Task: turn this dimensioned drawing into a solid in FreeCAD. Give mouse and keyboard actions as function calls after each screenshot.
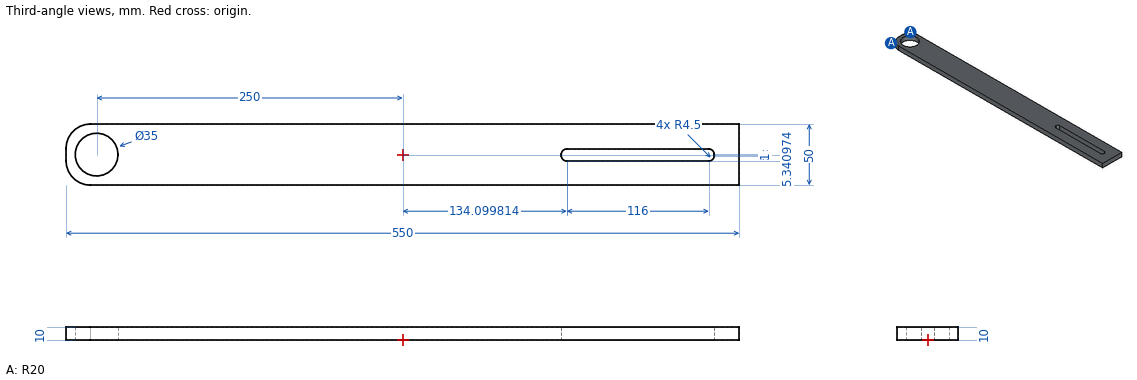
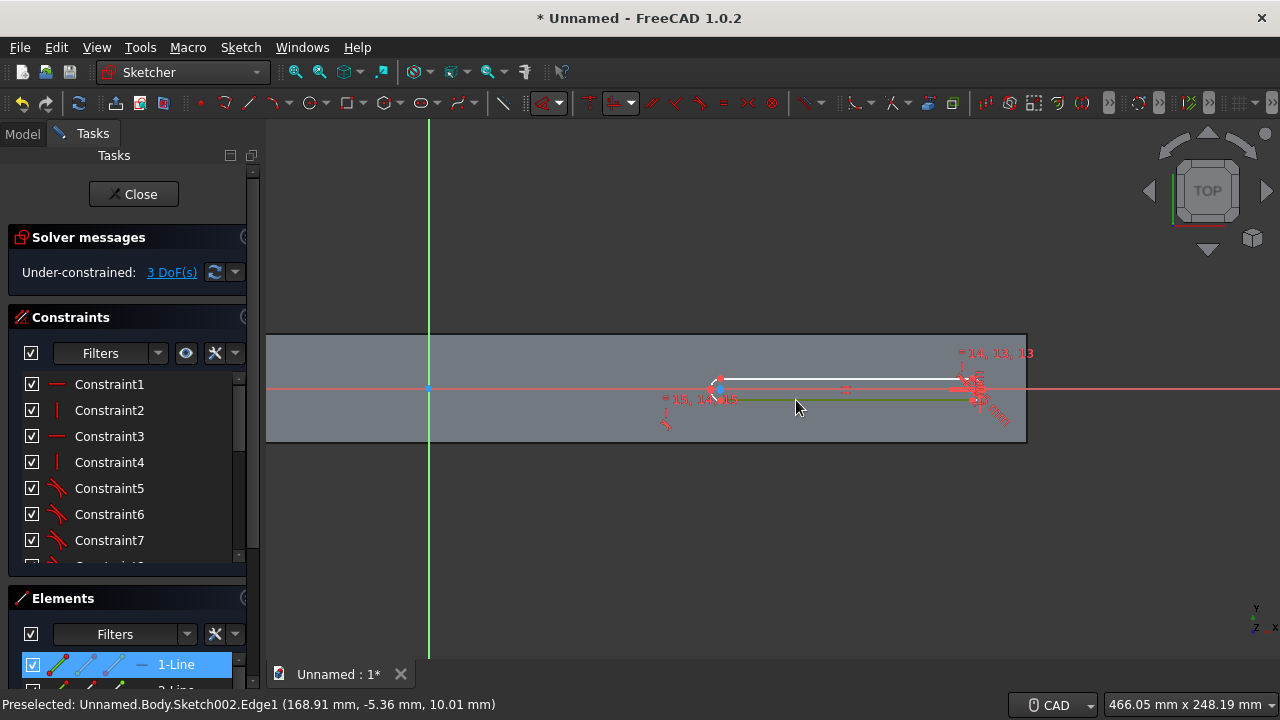
key(l)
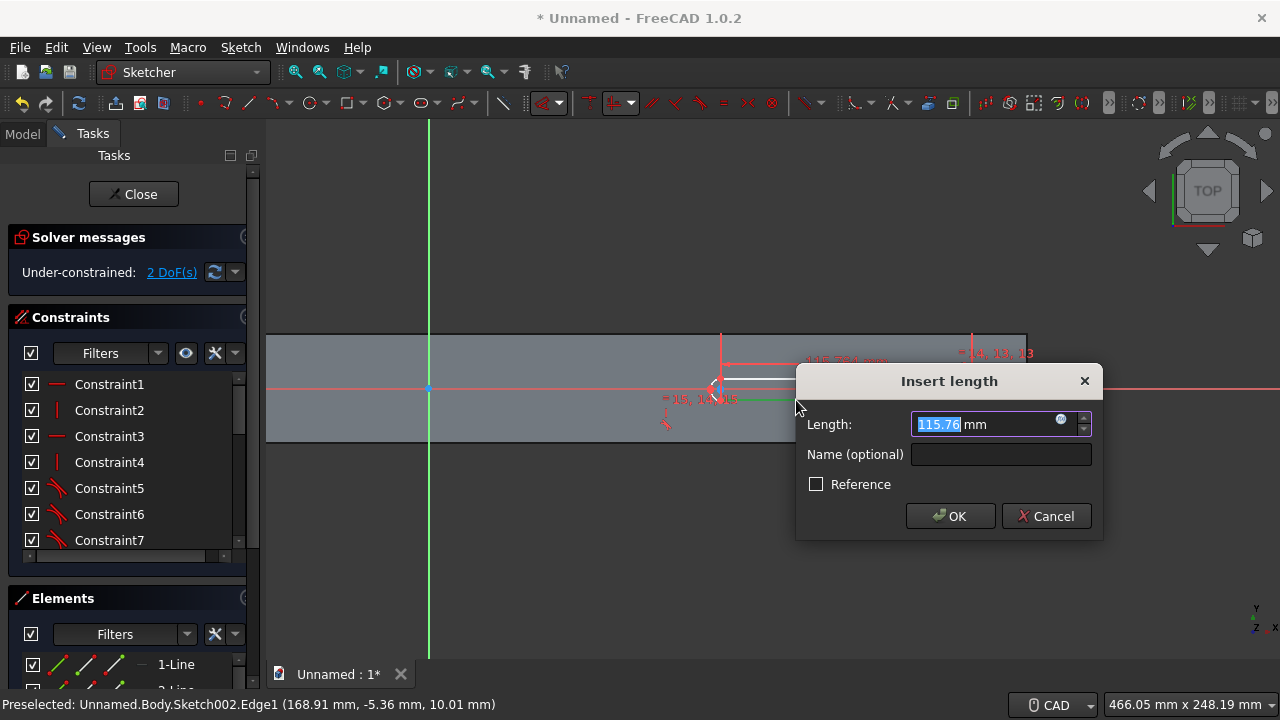
text(116)
key(Return)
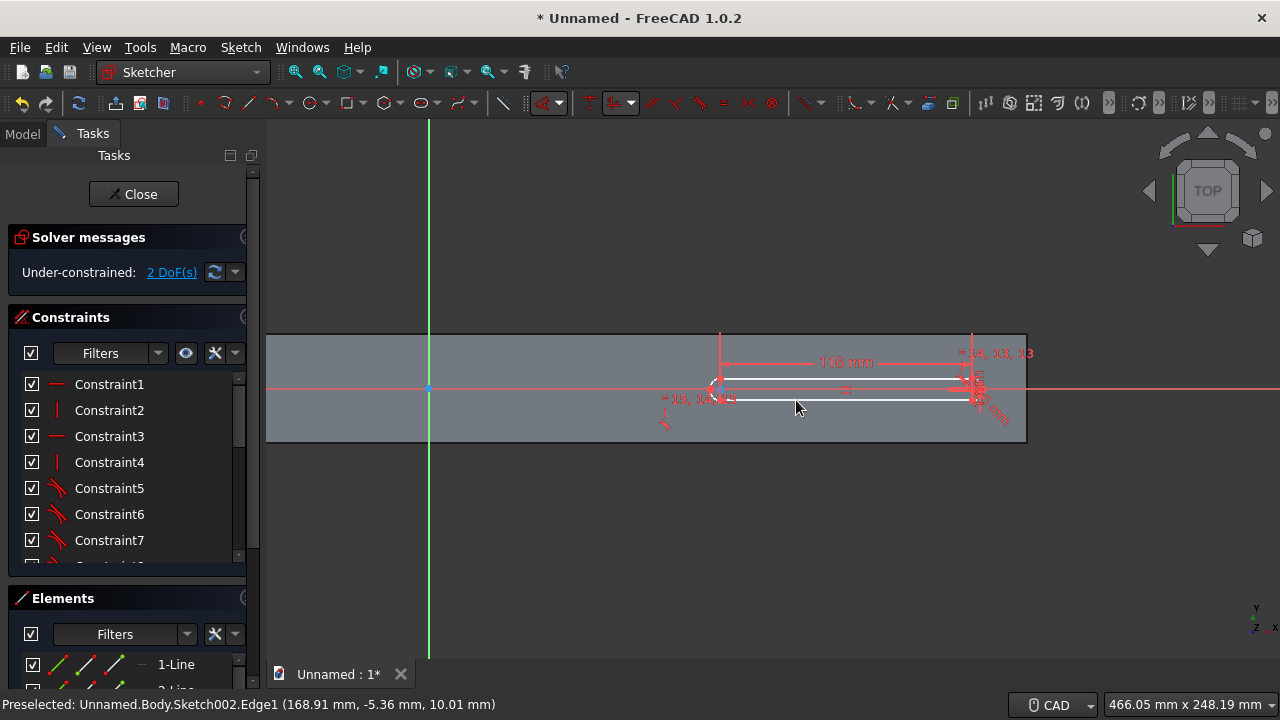
scroll(720, 400, up, 7)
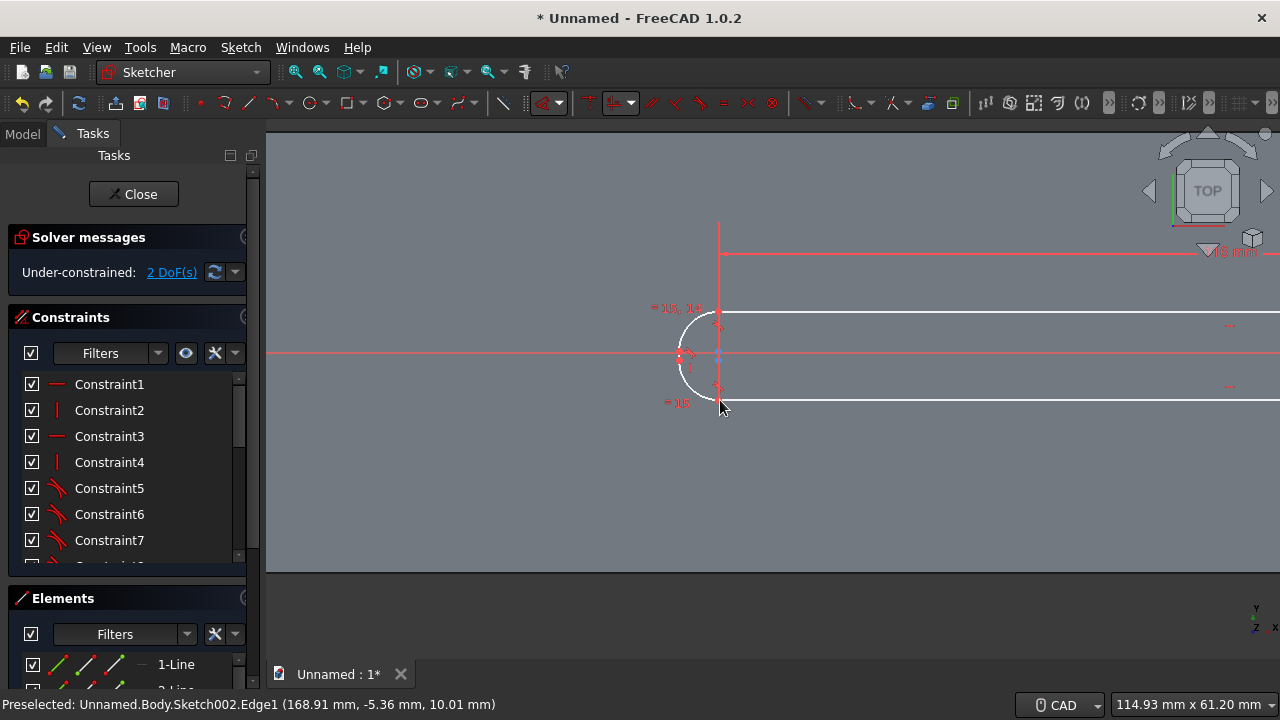
click(719, 400)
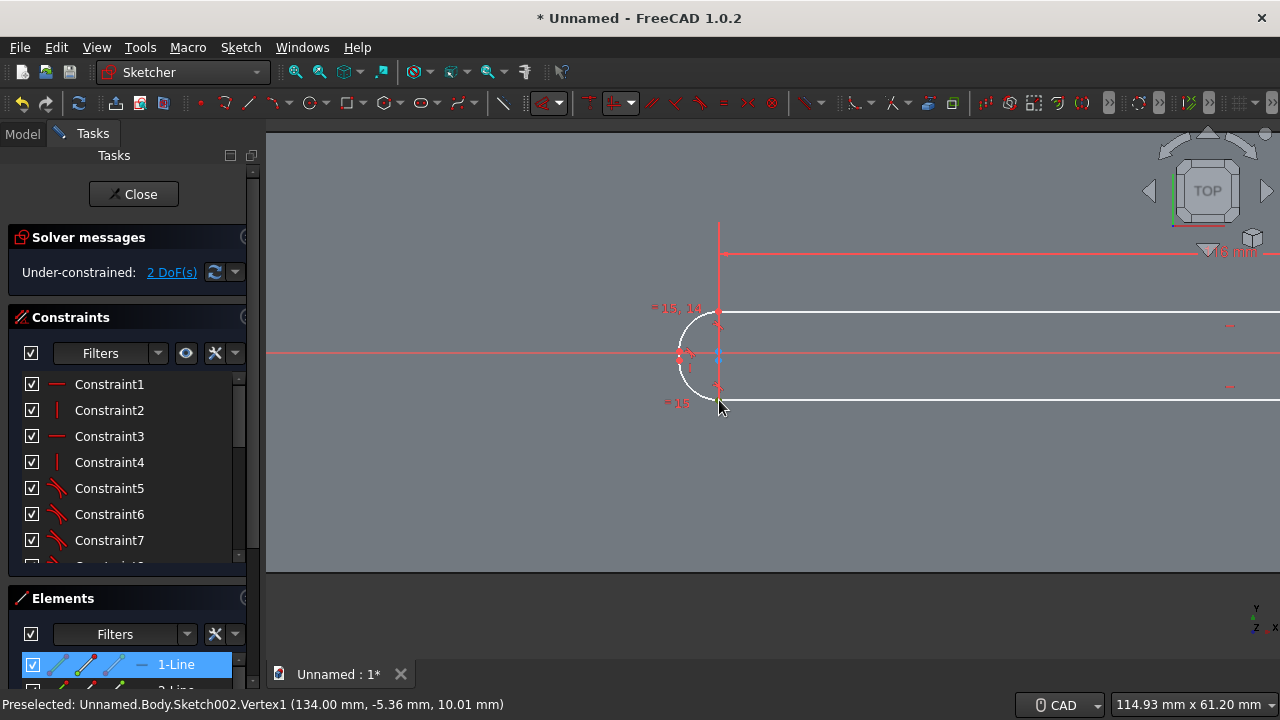
key(i)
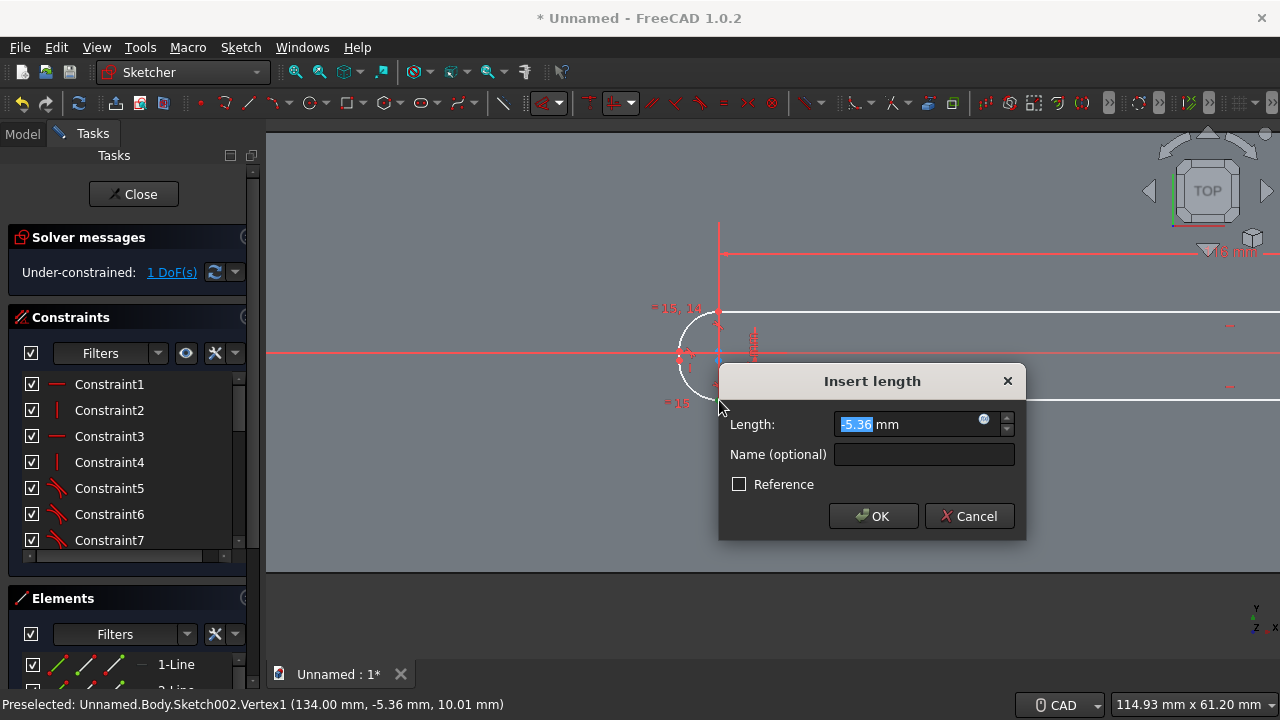
text(-5.340974)
key(Return)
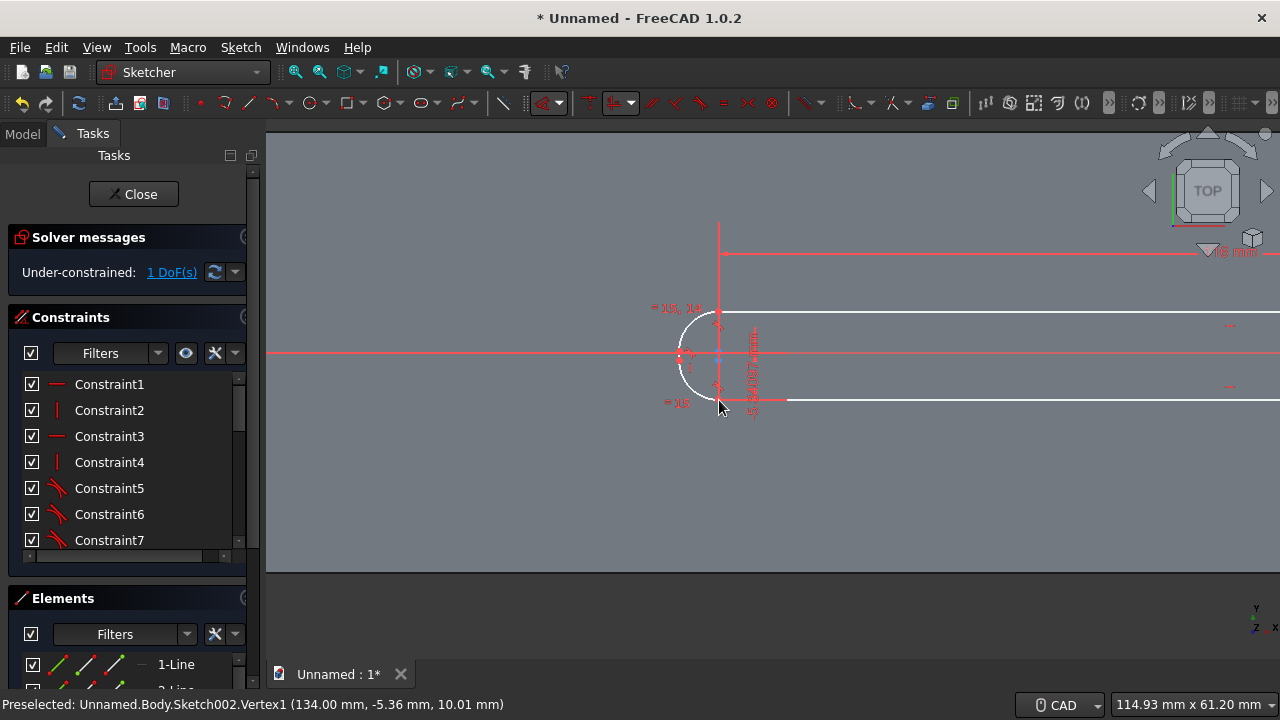
scroll(719, 400, down, 7)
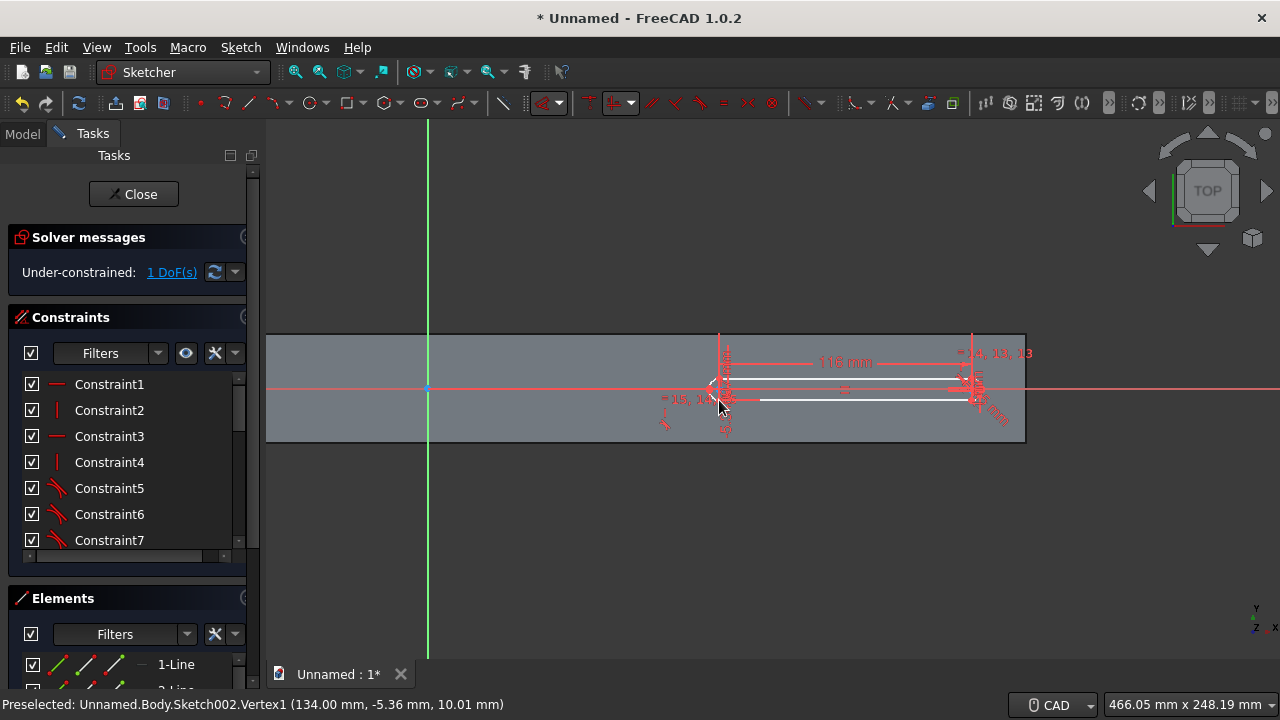
scroll(719, 400, up, 2)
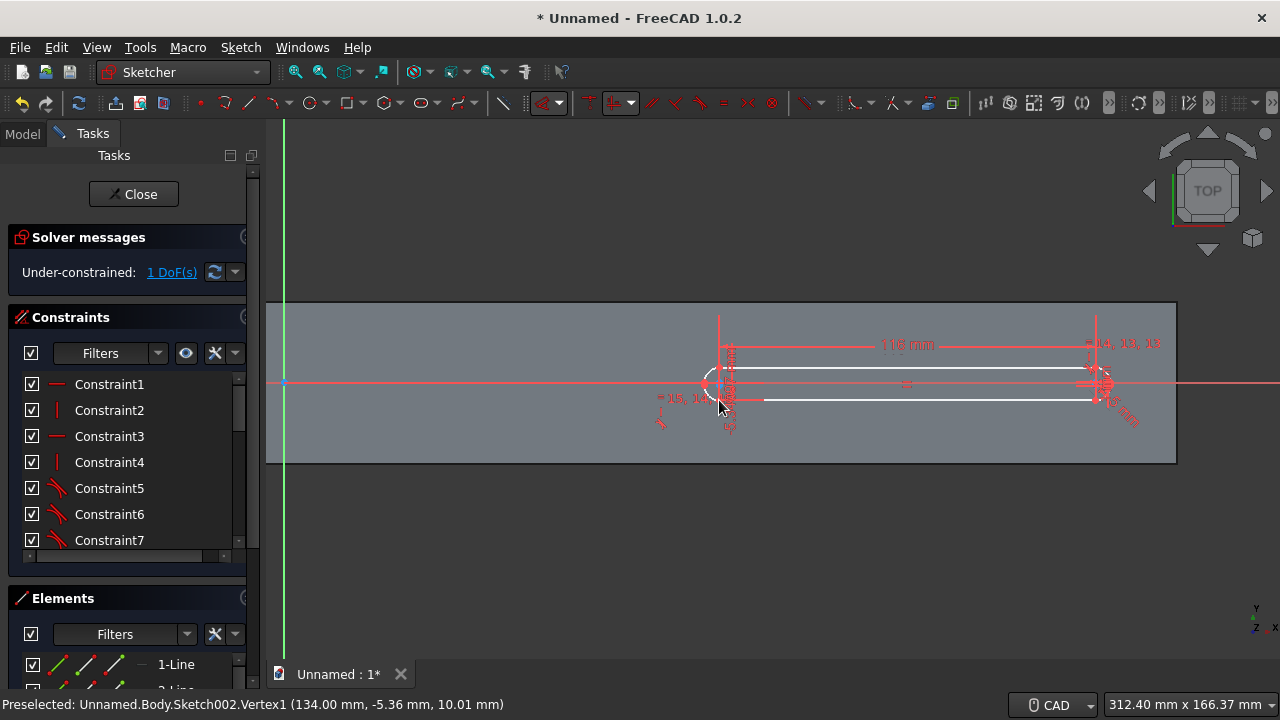
scroll(719, 400, up, 4)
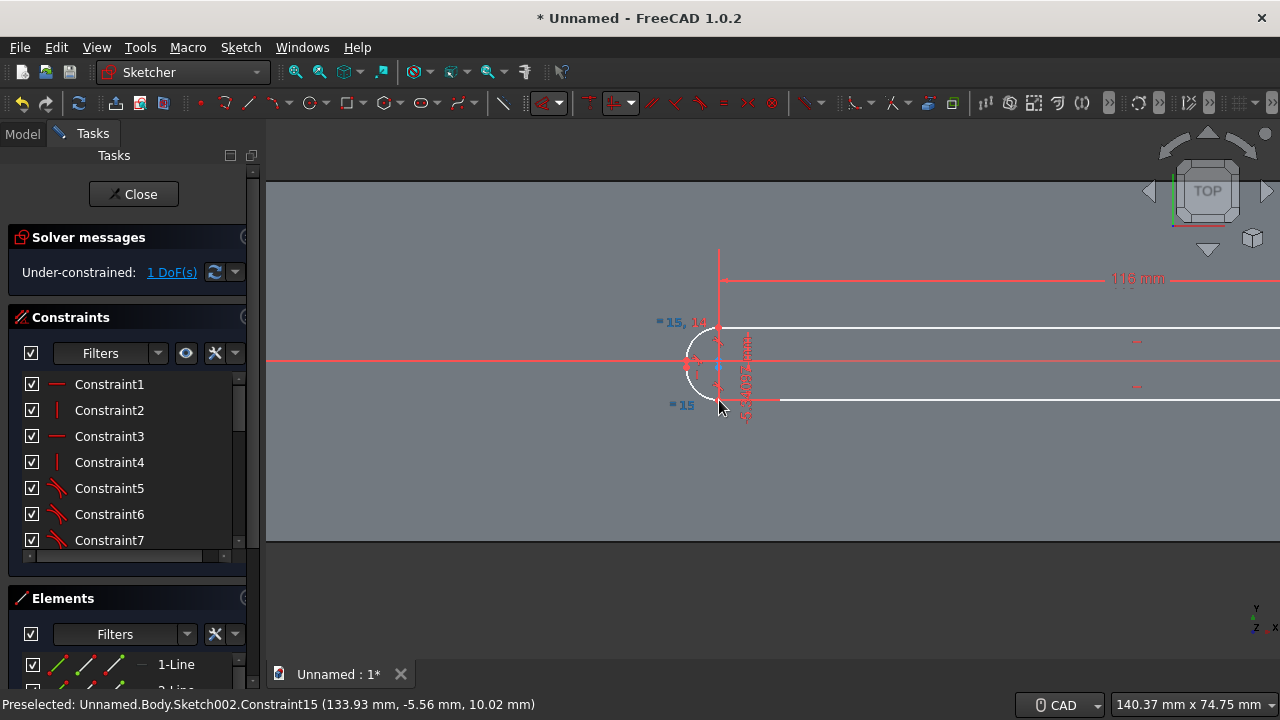
click(719, 400)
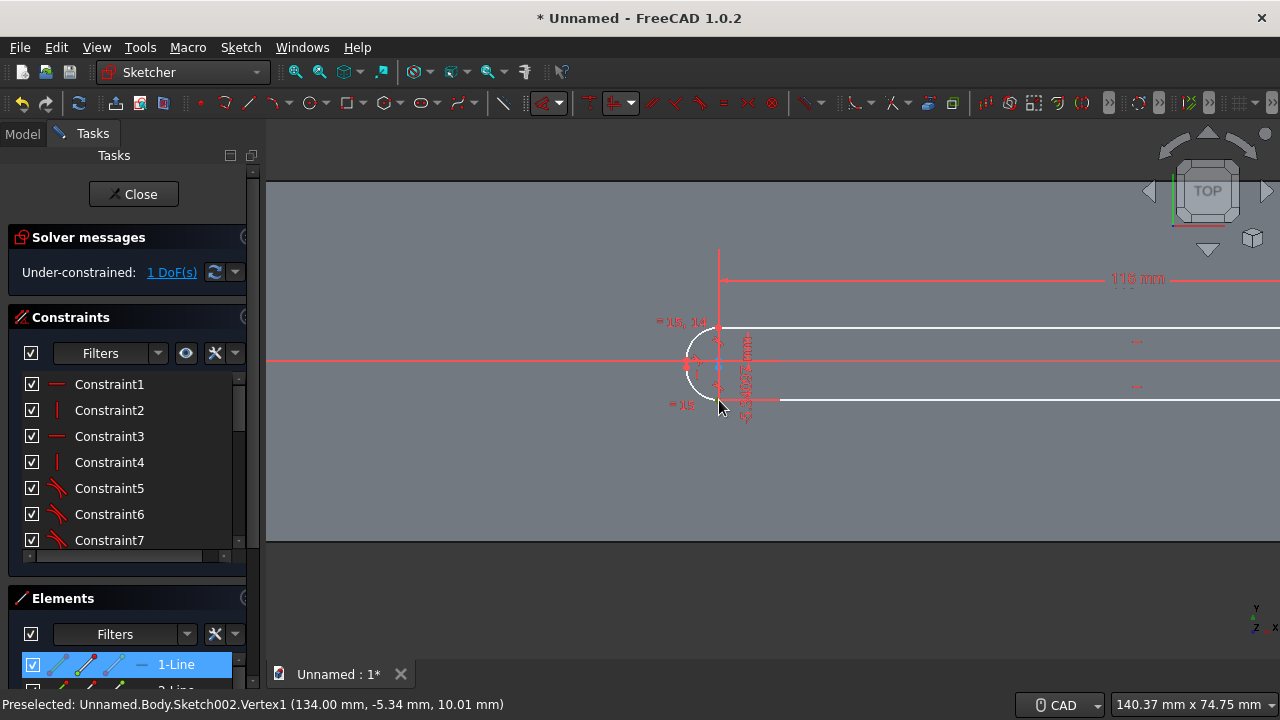
key(l)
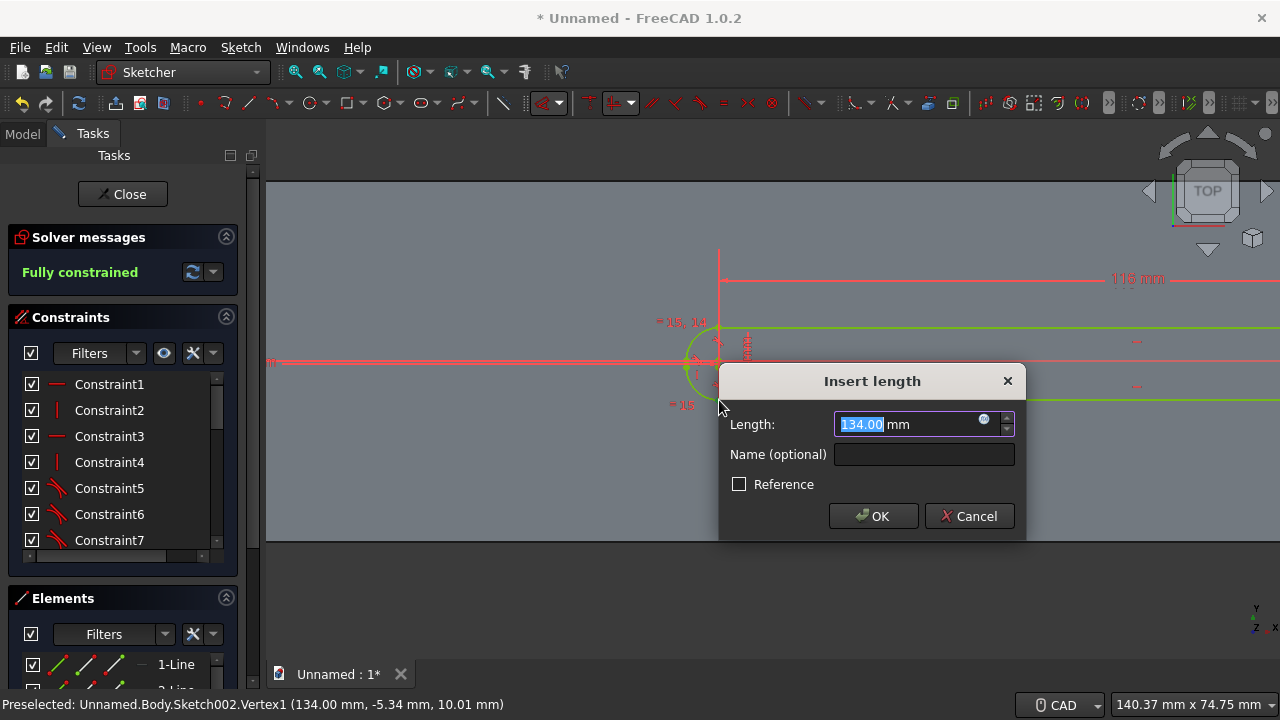
text(134.099814)
key(Return)